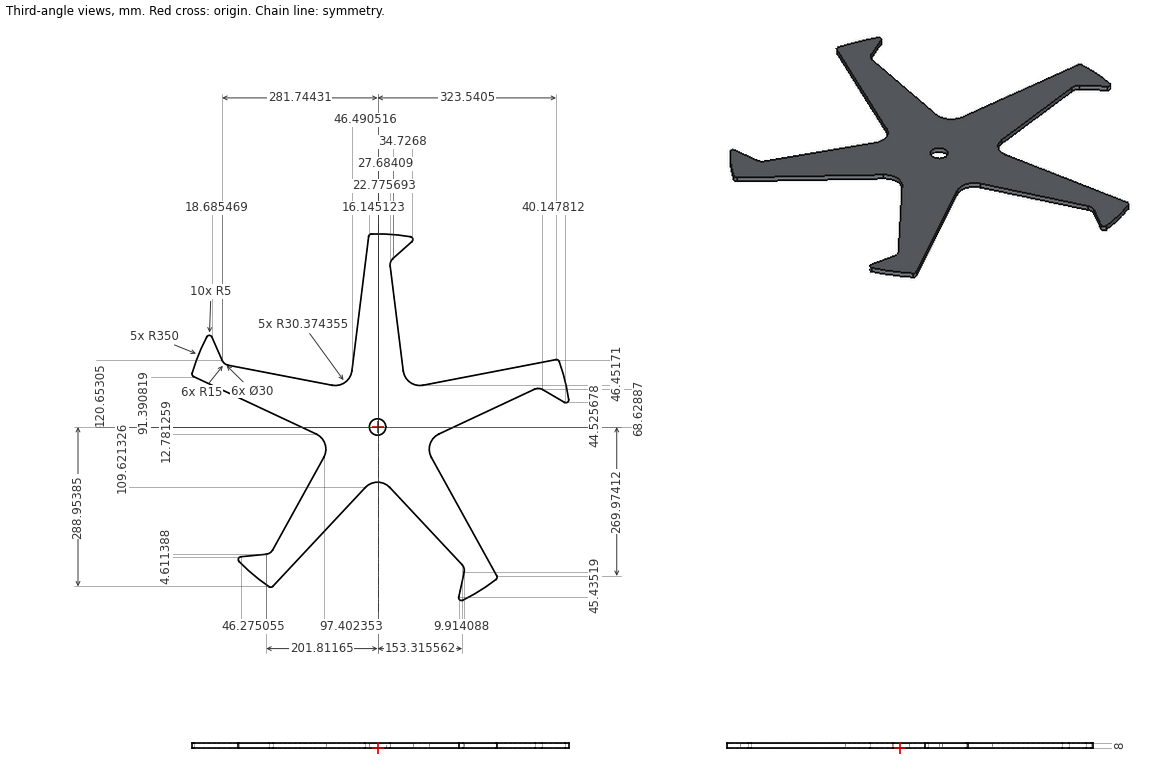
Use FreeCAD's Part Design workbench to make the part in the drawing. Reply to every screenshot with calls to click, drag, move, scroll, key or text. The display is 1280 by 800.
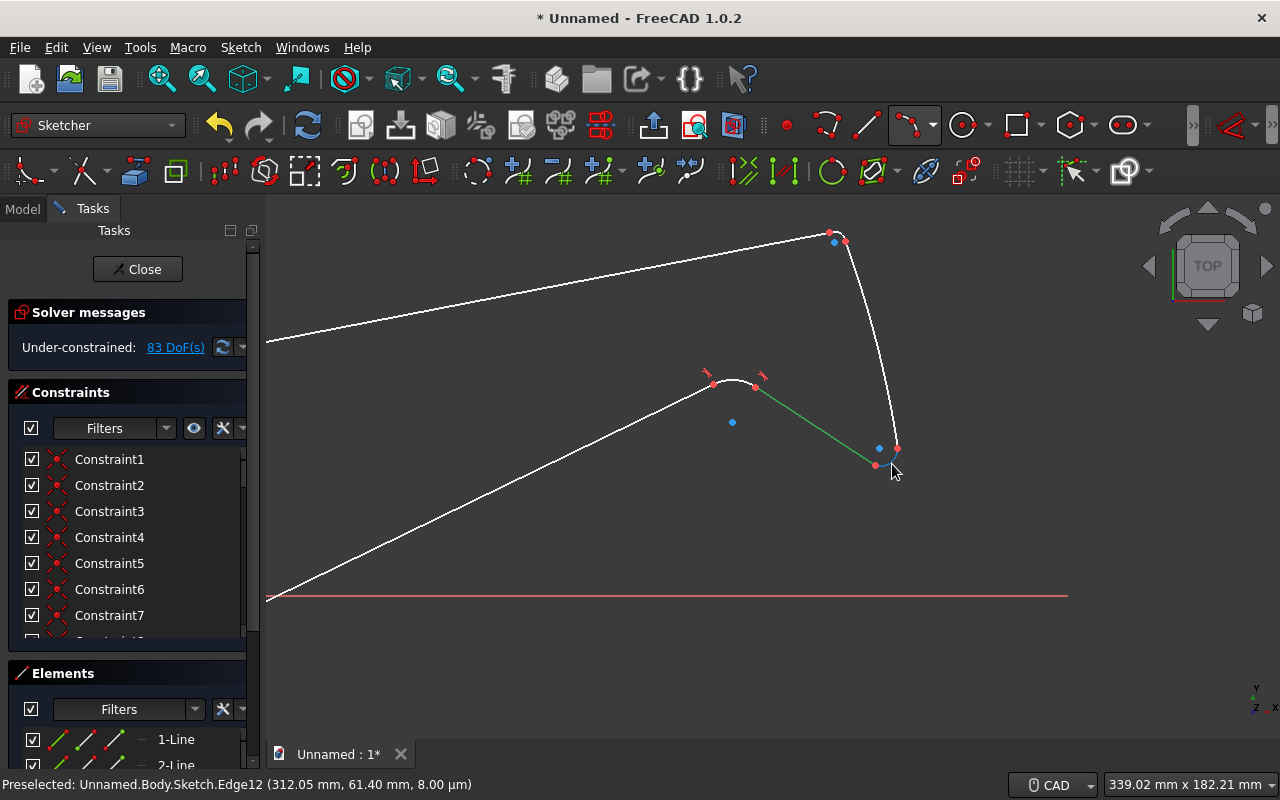
click(891, 463)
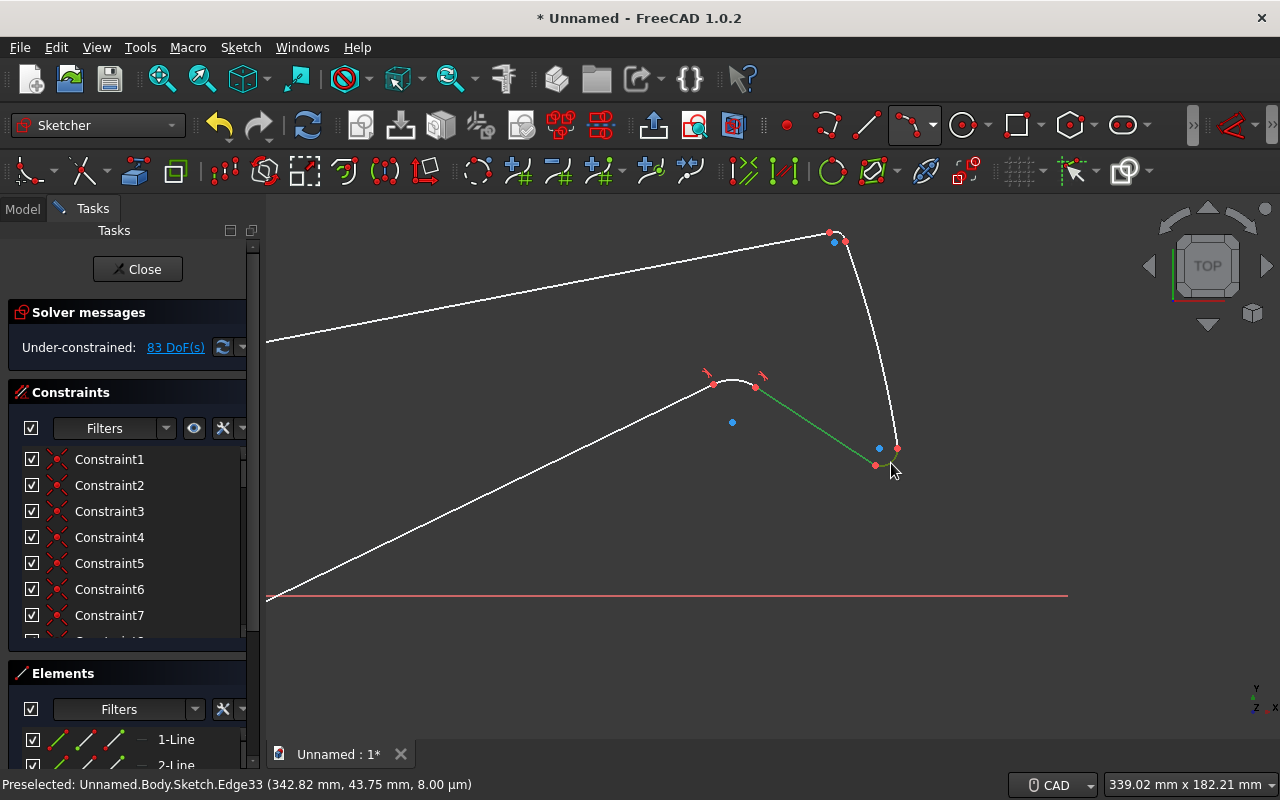
key(t)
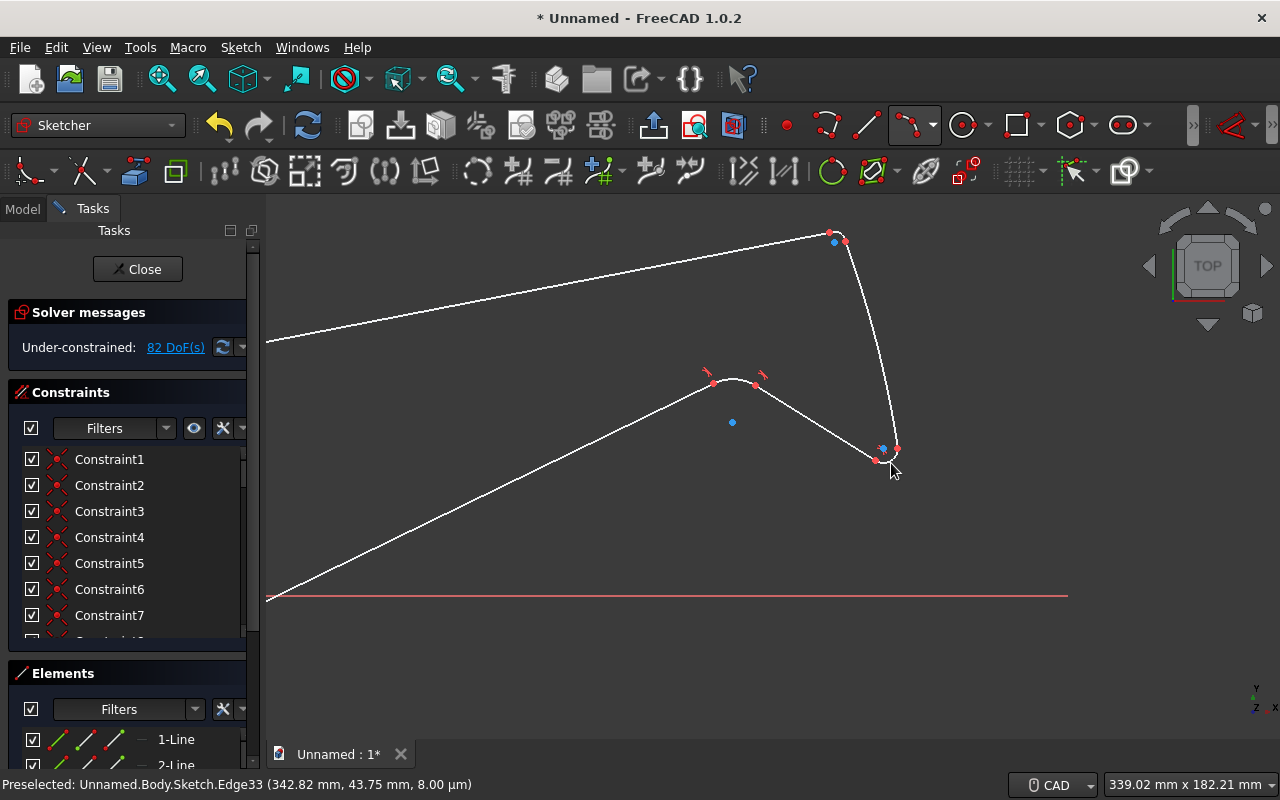
scroll(868, 451, down, 9)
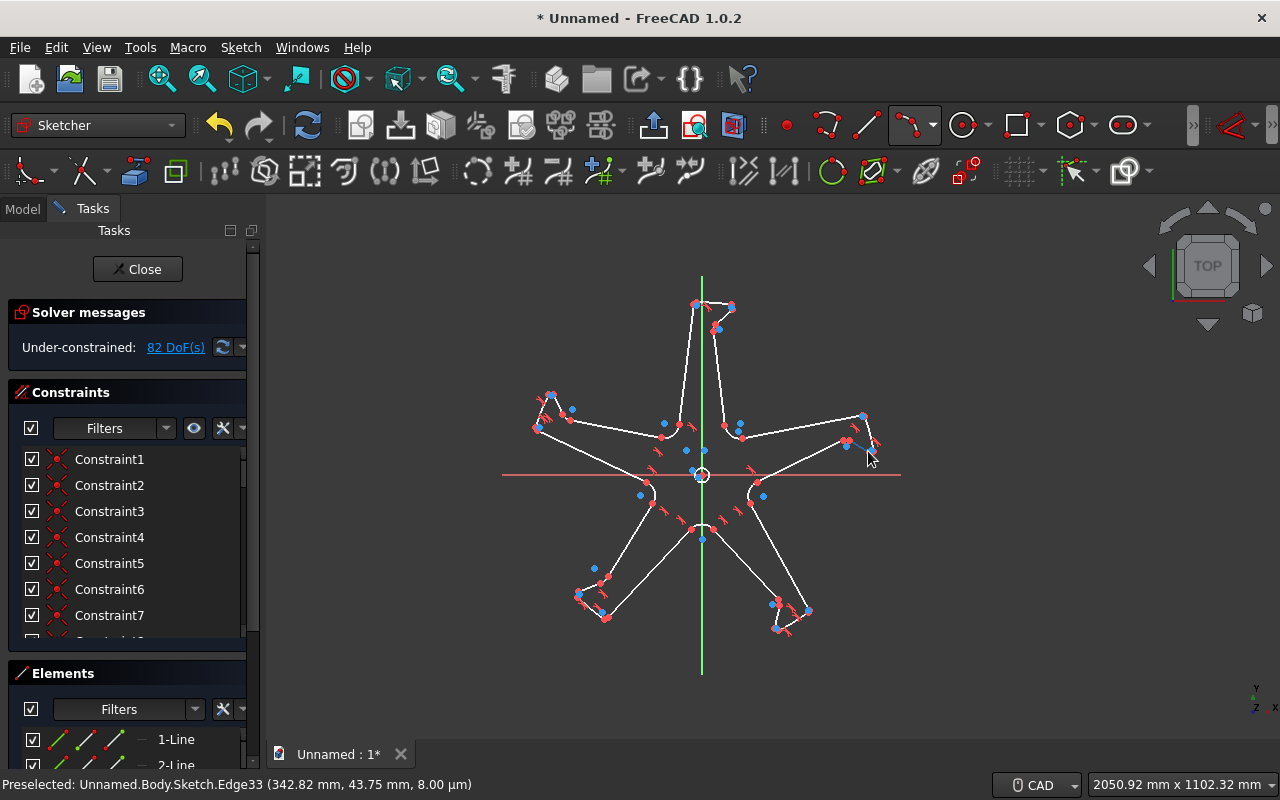
click(826, 422)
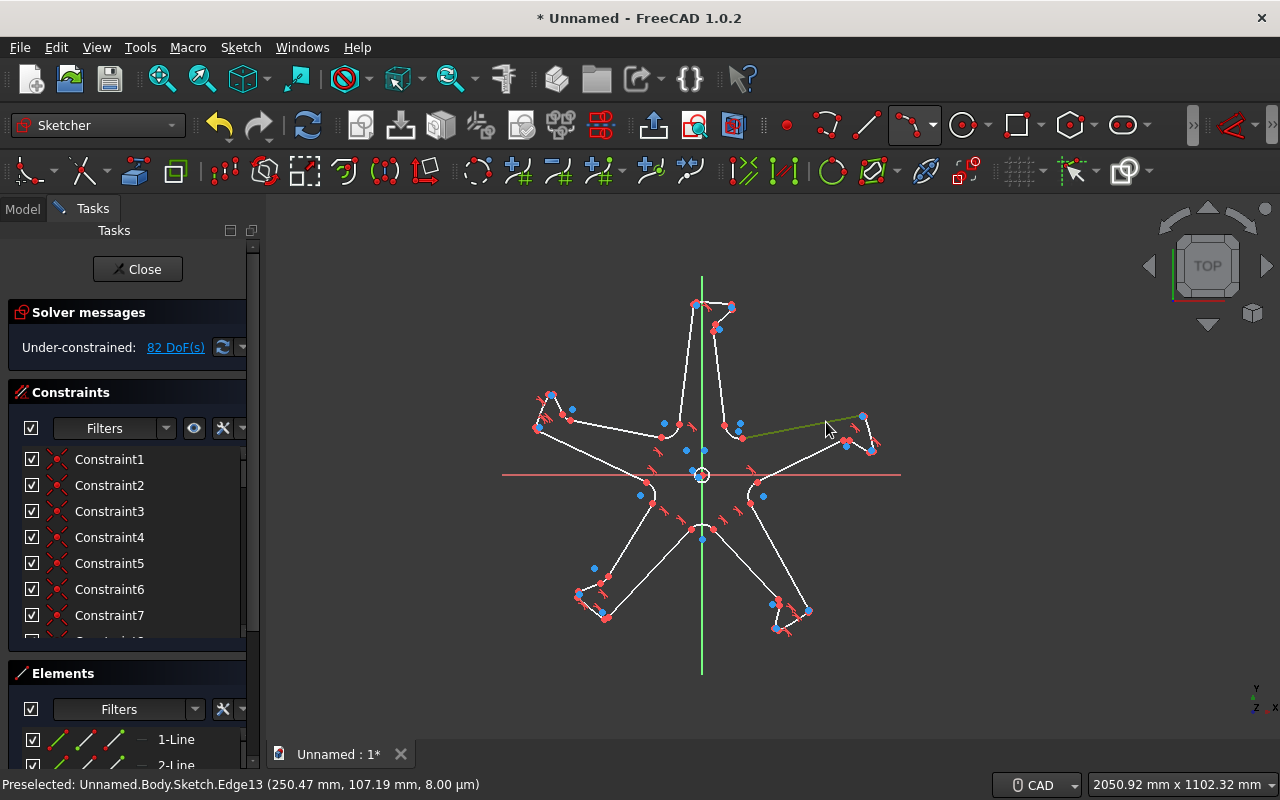
scroll(864, 415, up, 11)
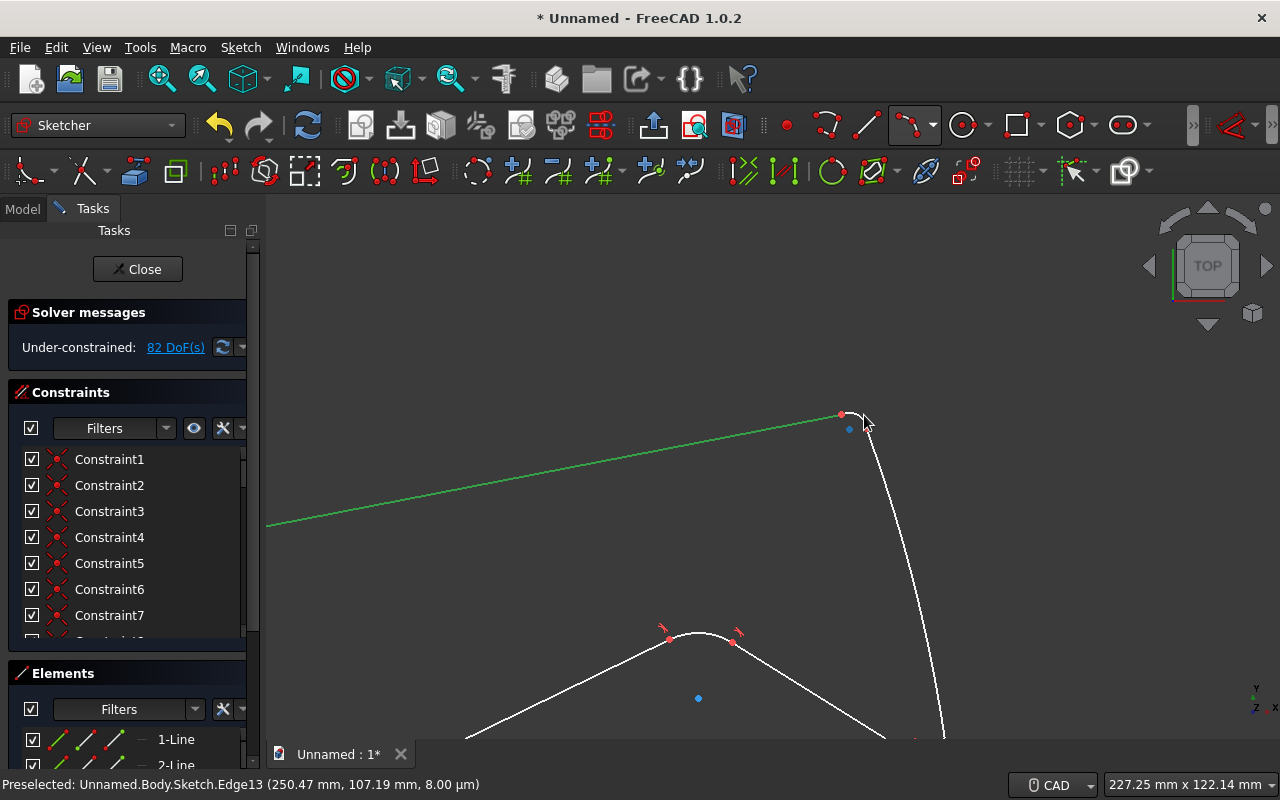
click(858, 415)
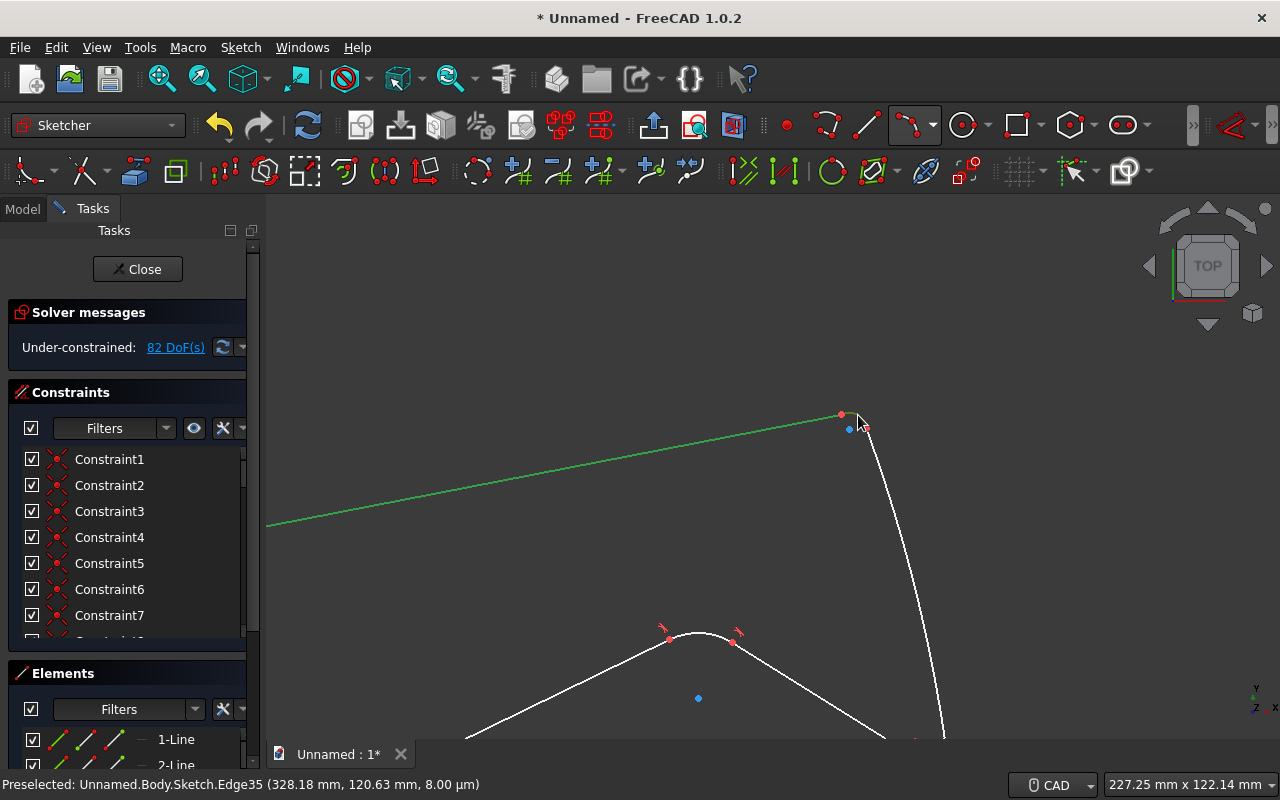
key(t)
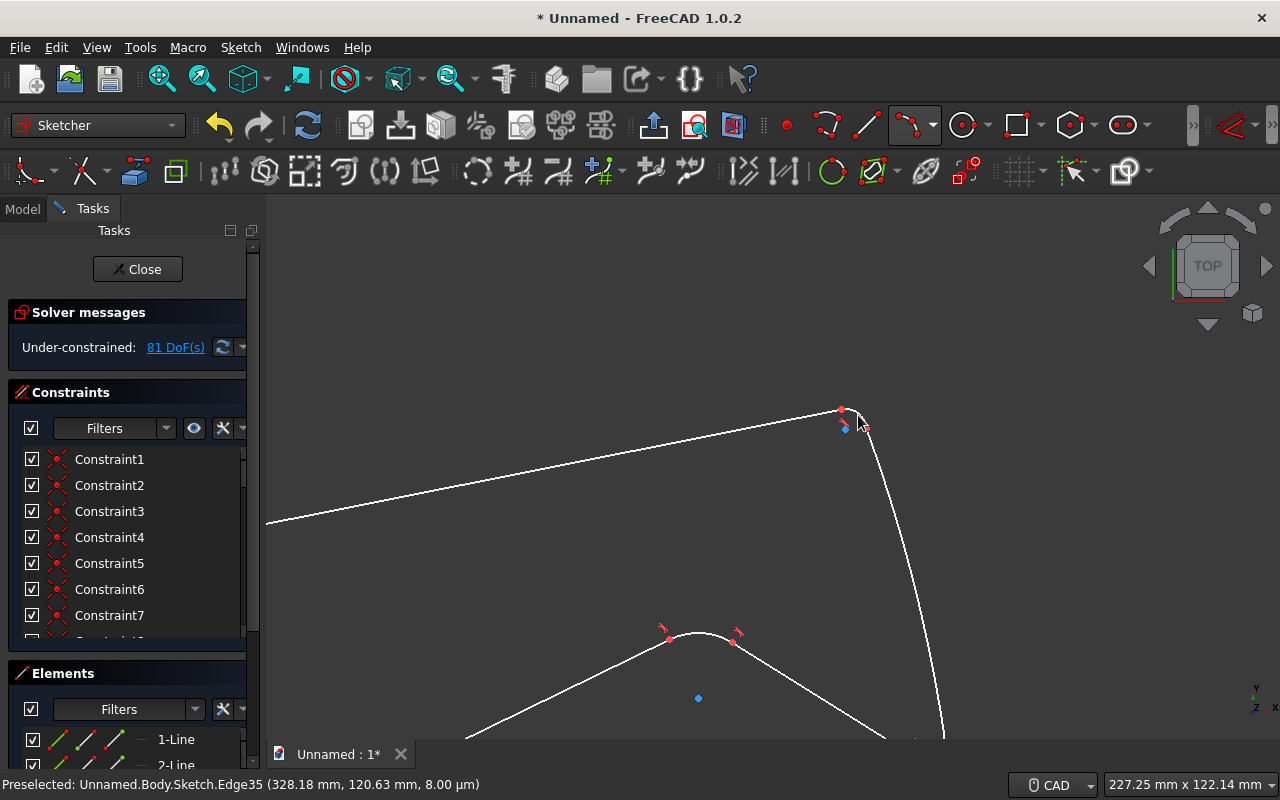
scroll(864, 415, down, 11)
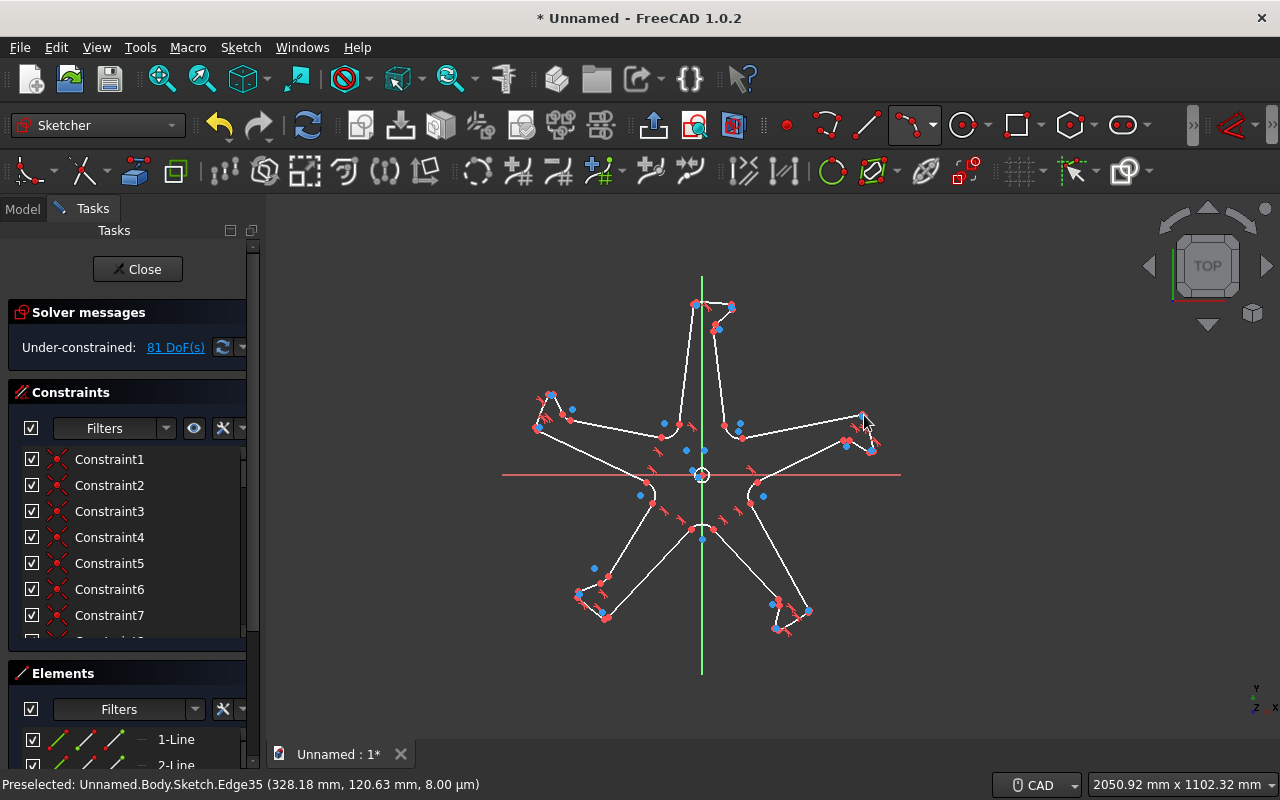
click(826, 422)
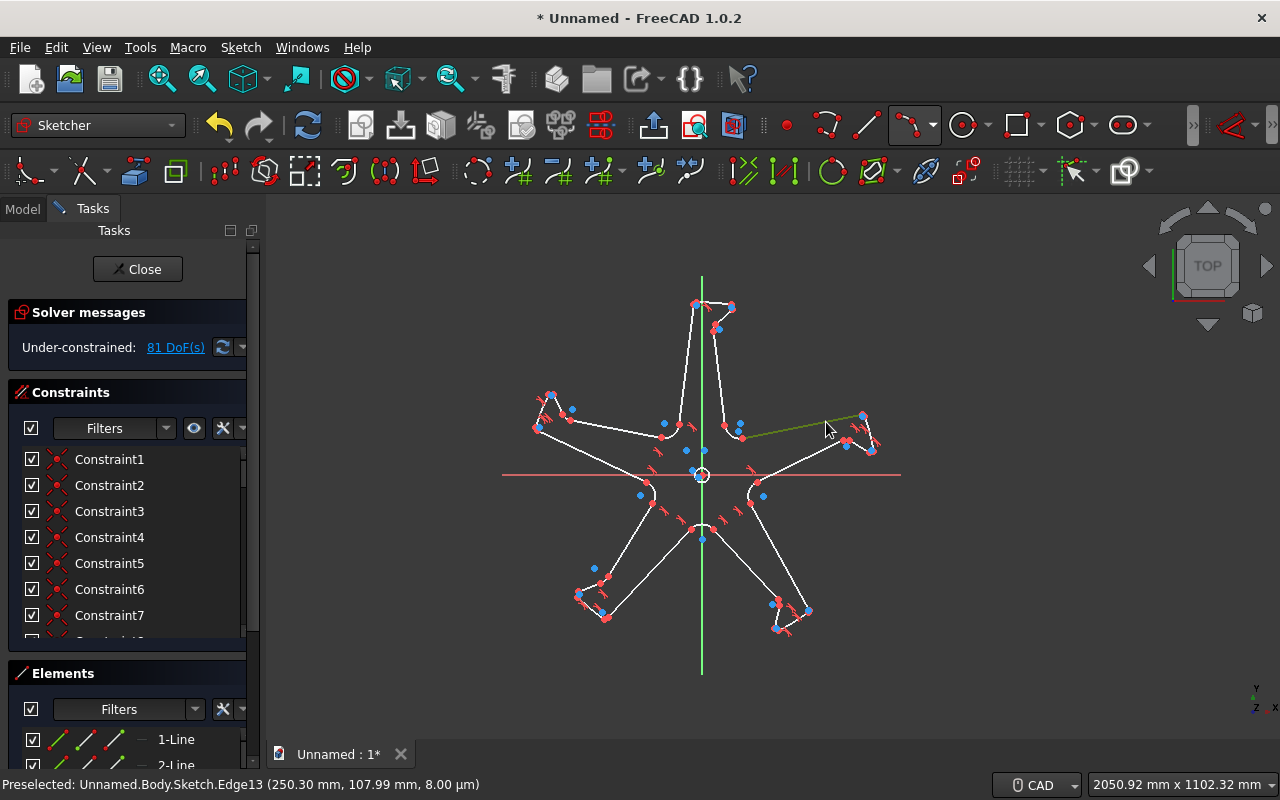
click(731, 436)